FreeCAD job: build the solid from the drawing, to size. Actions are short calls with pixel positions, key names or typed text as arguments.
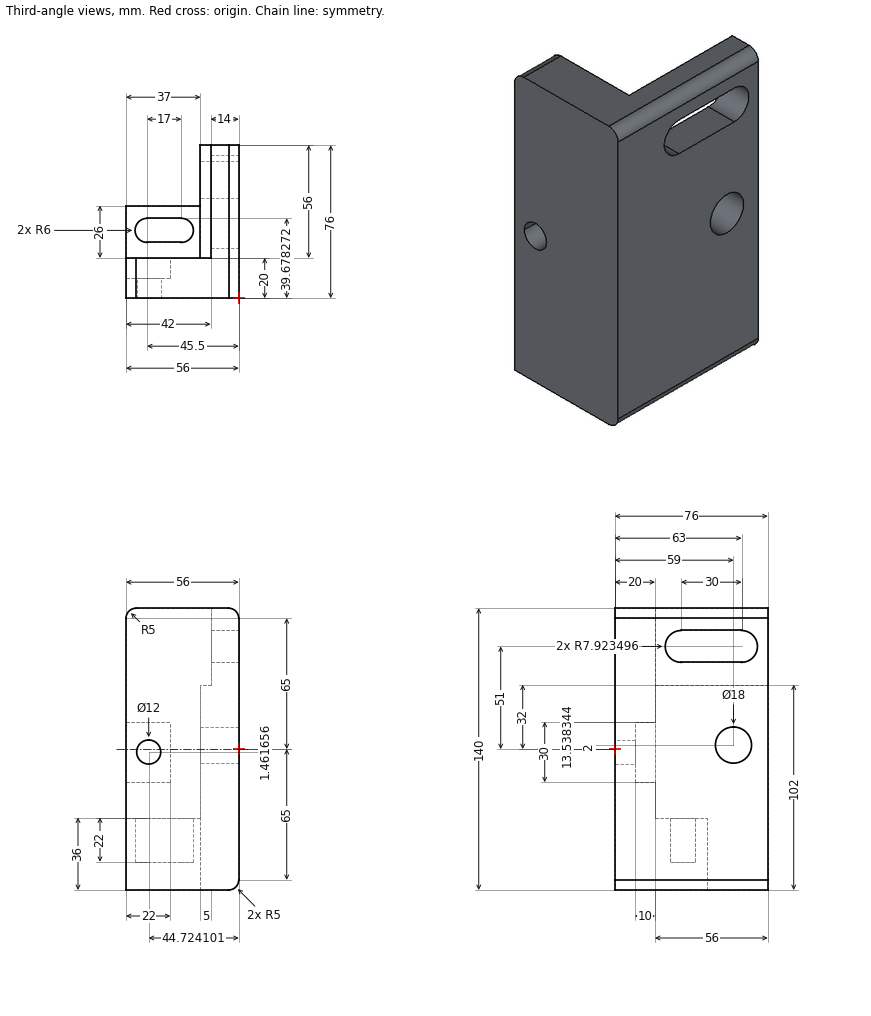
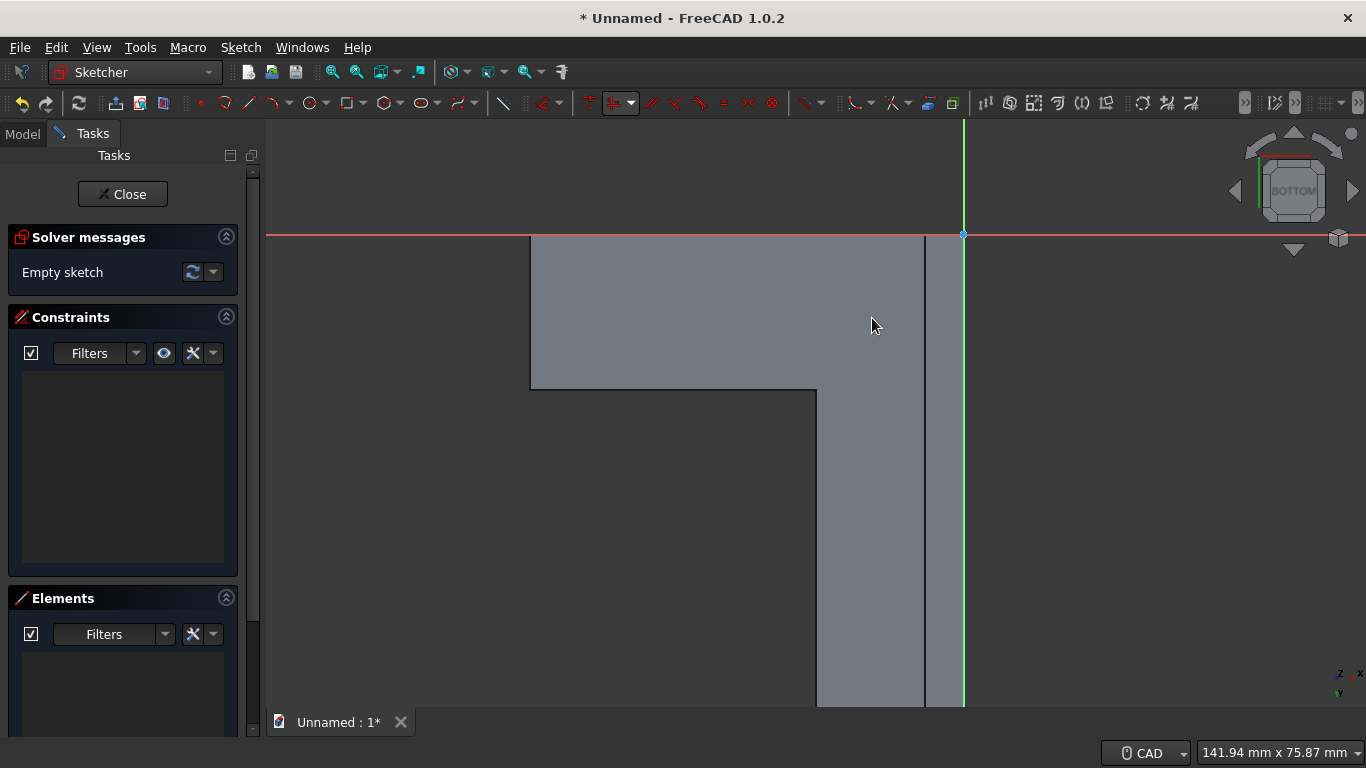
key(g)
key(r)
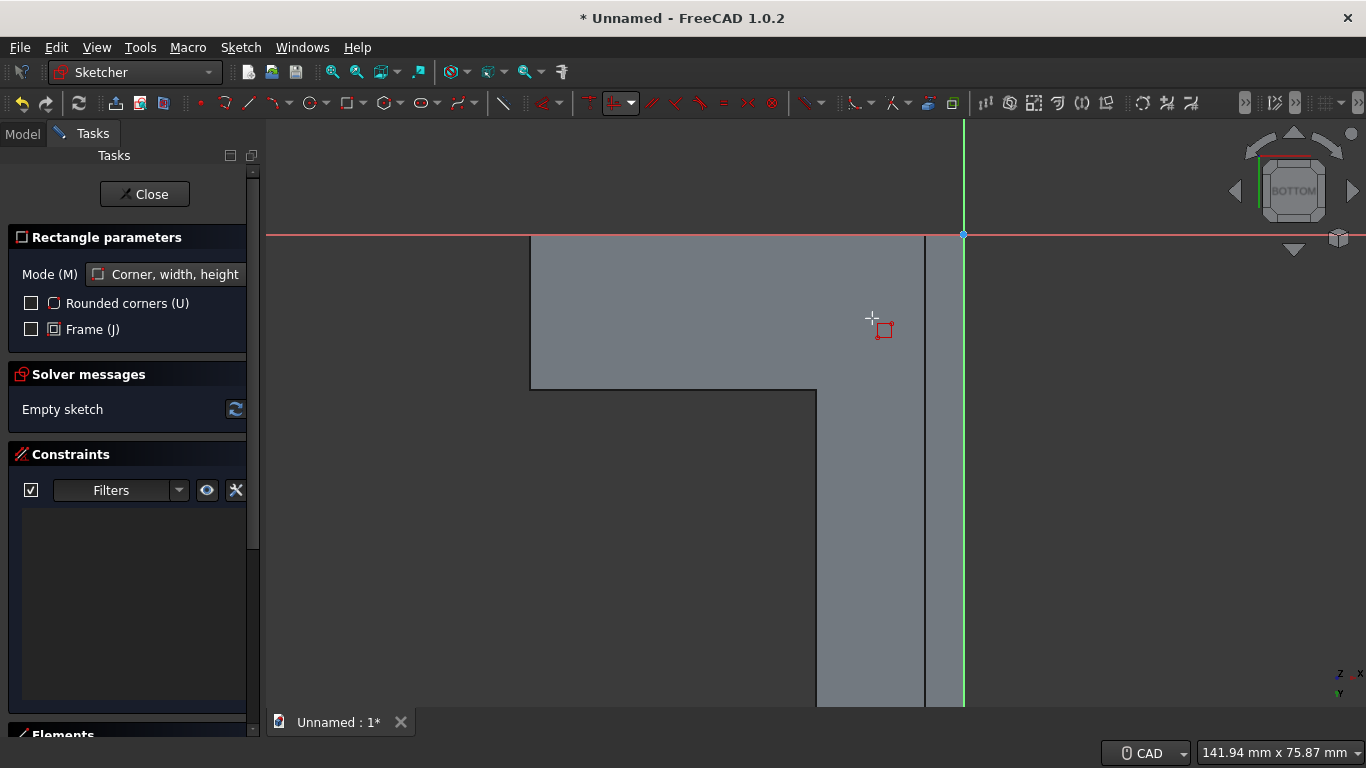
click(530, 390)
click(816, 591)
key(Escape)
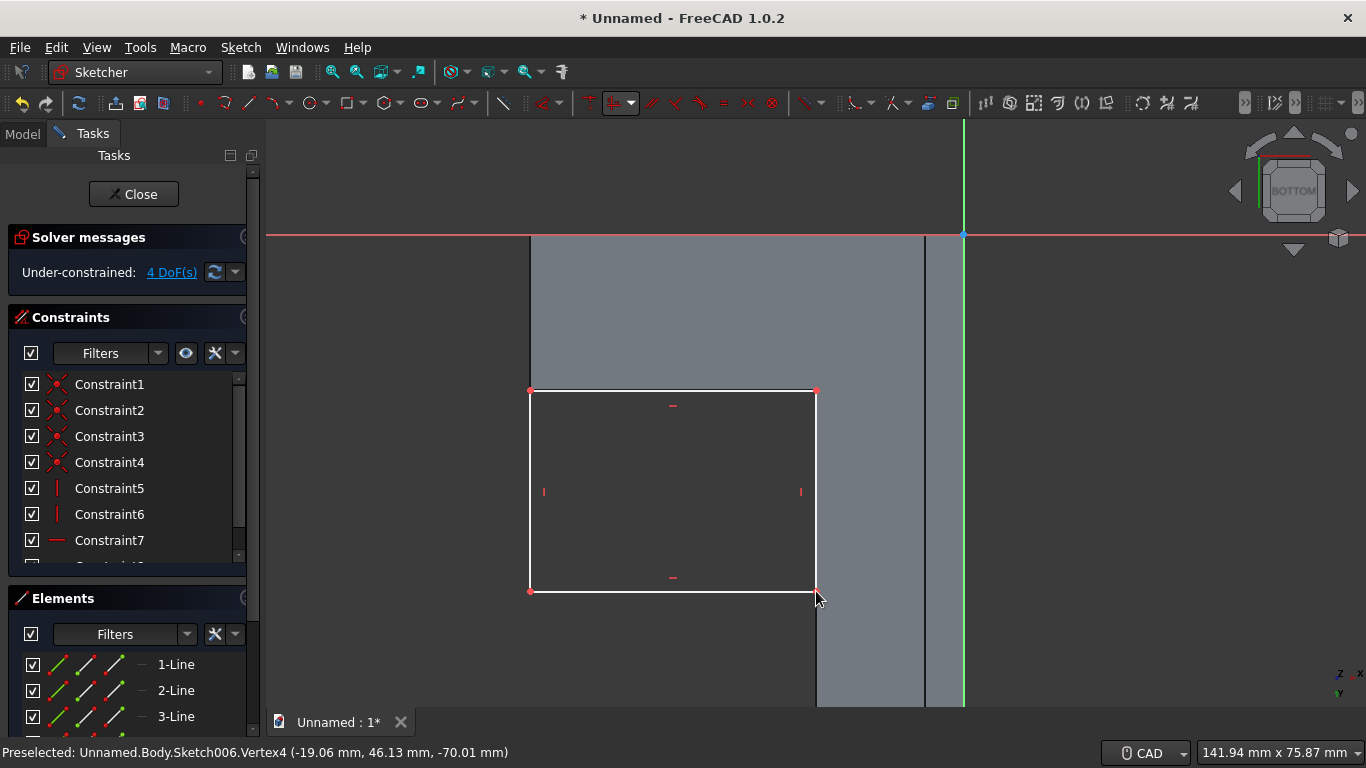
key(d)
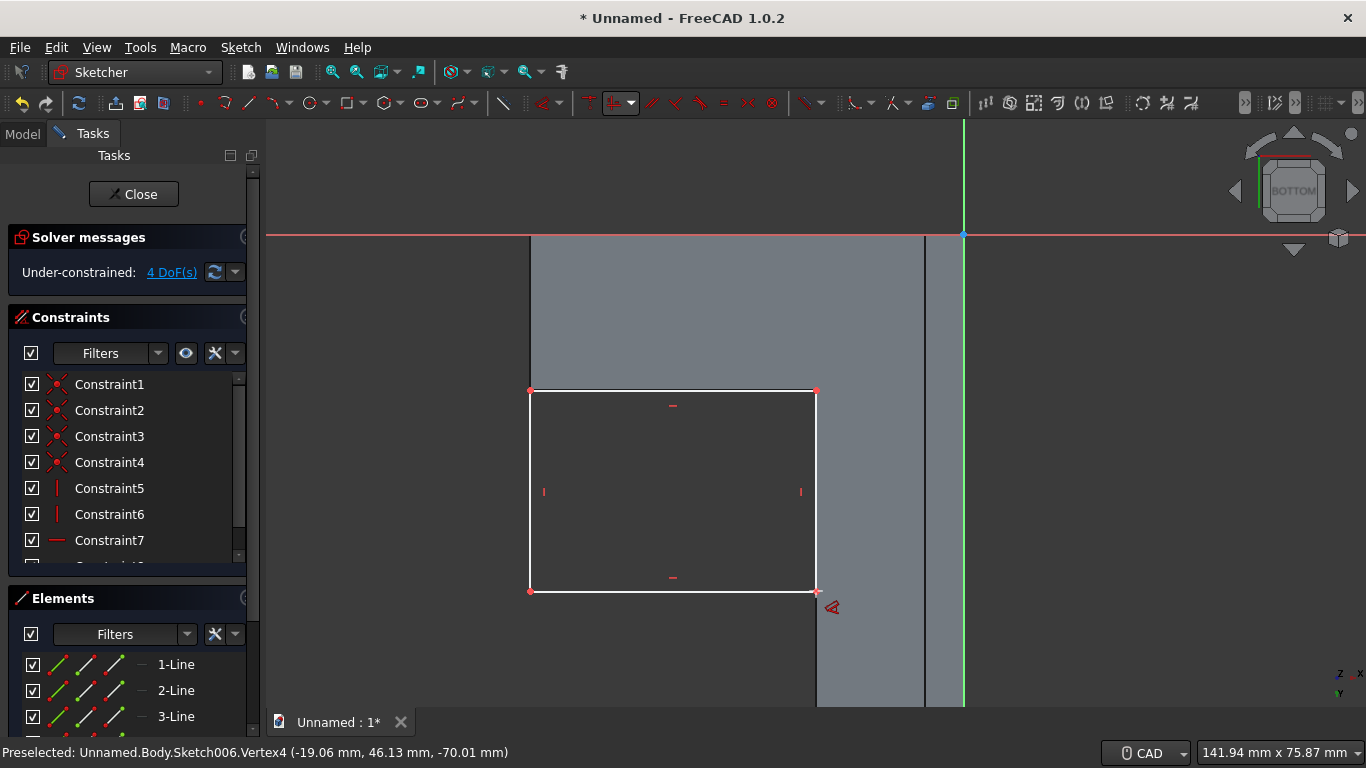
click(530, 451)
click(496, 491)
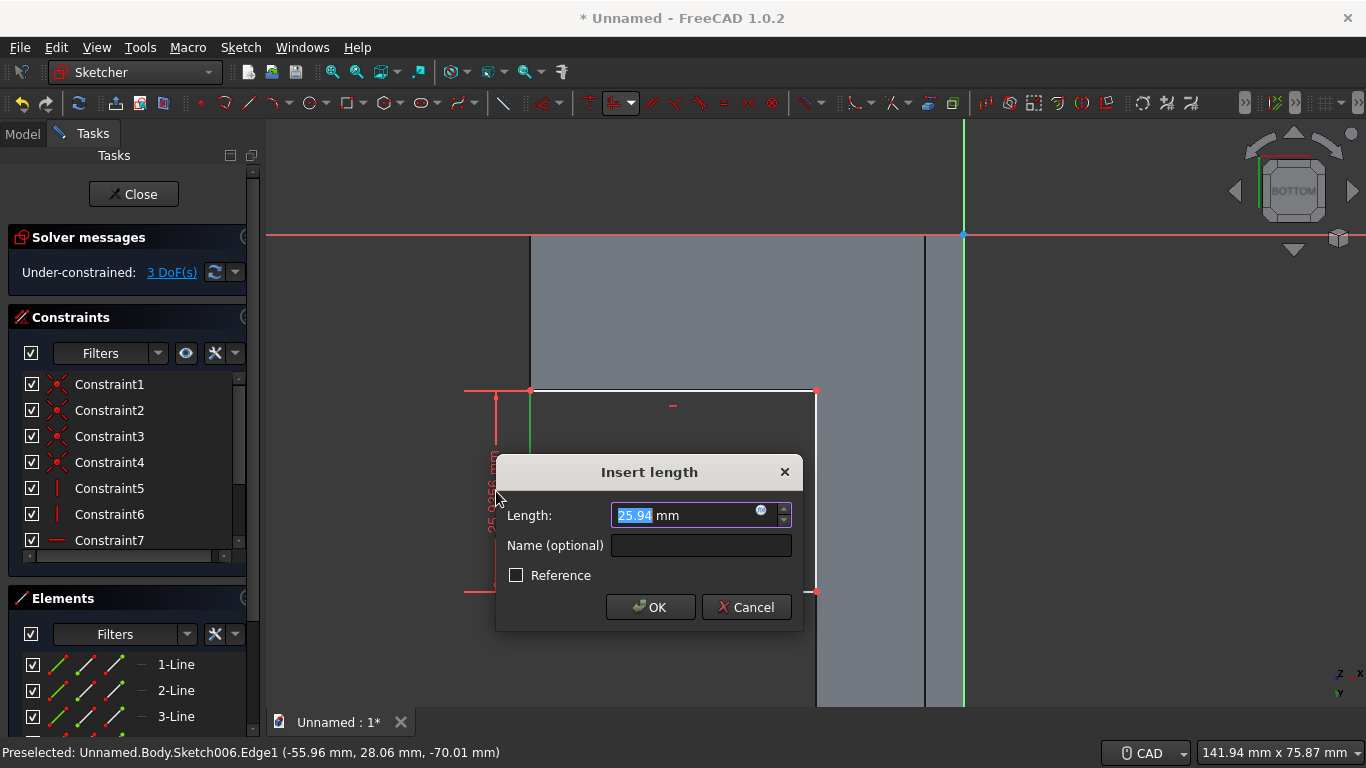
text(26)
key(Return)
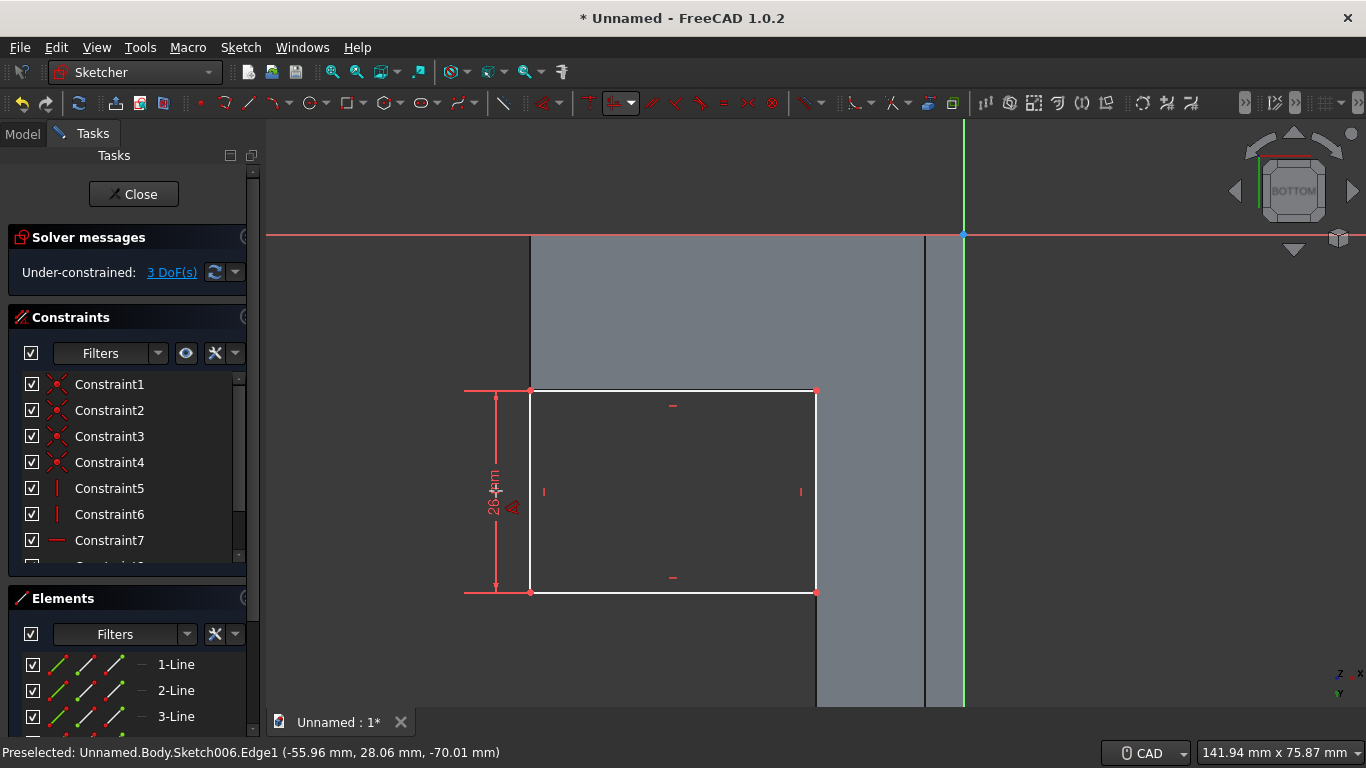
click(616, 592)
click(673, 626)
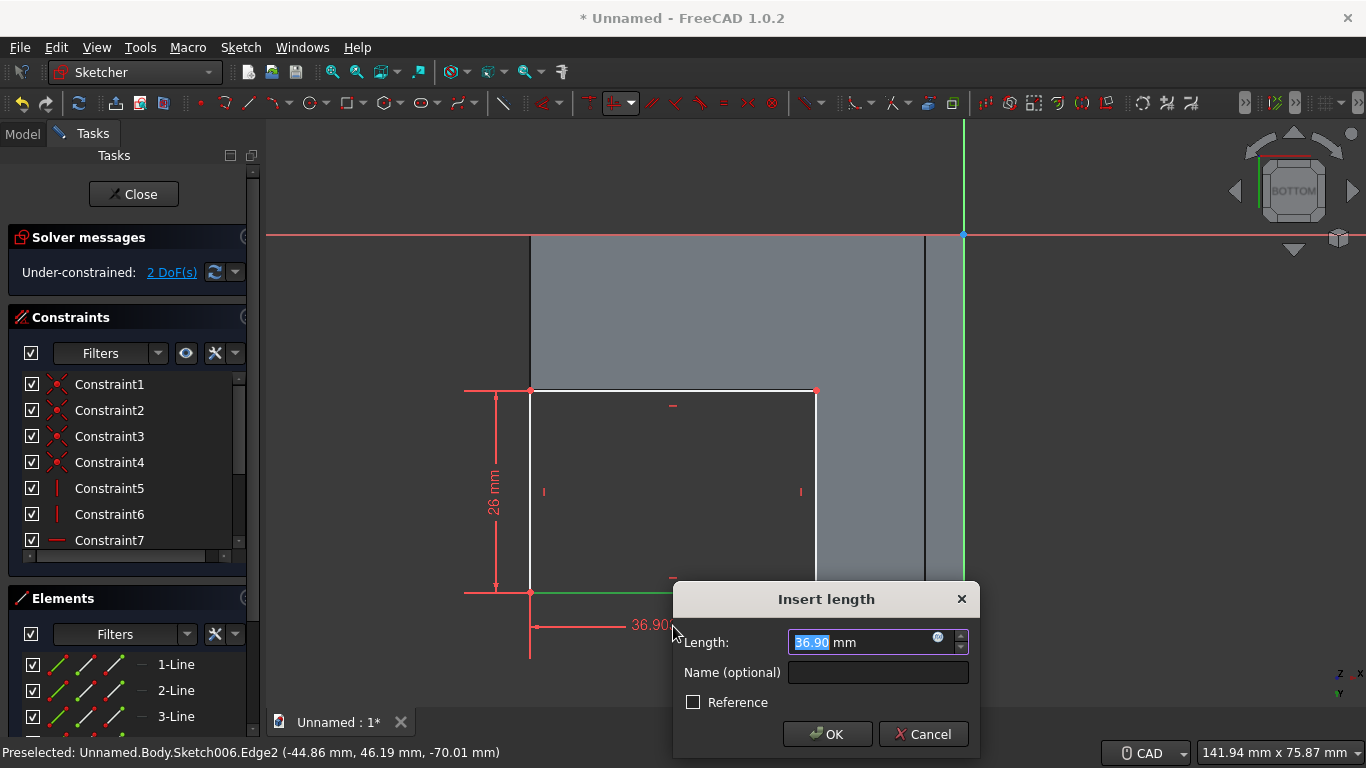
text(37)
key(Return)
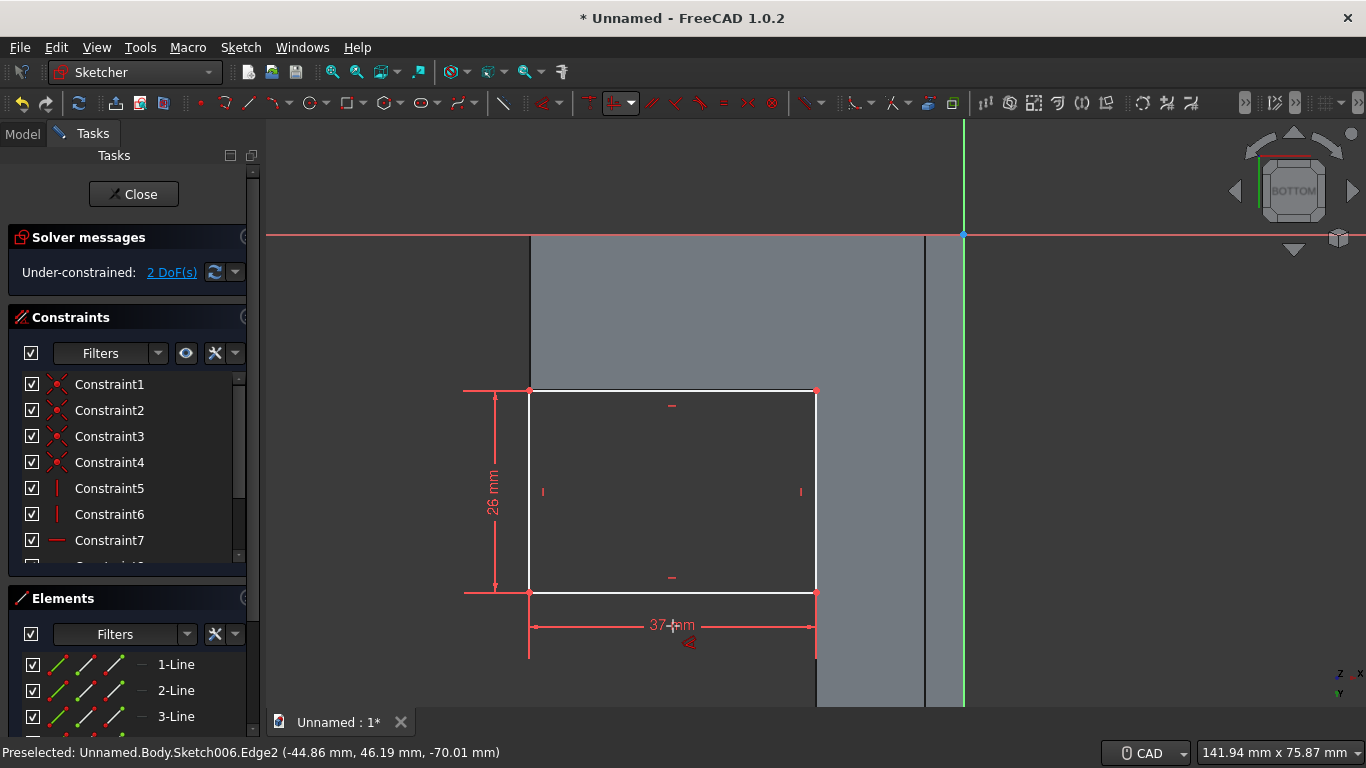
click(529, 391)
click(746, 201)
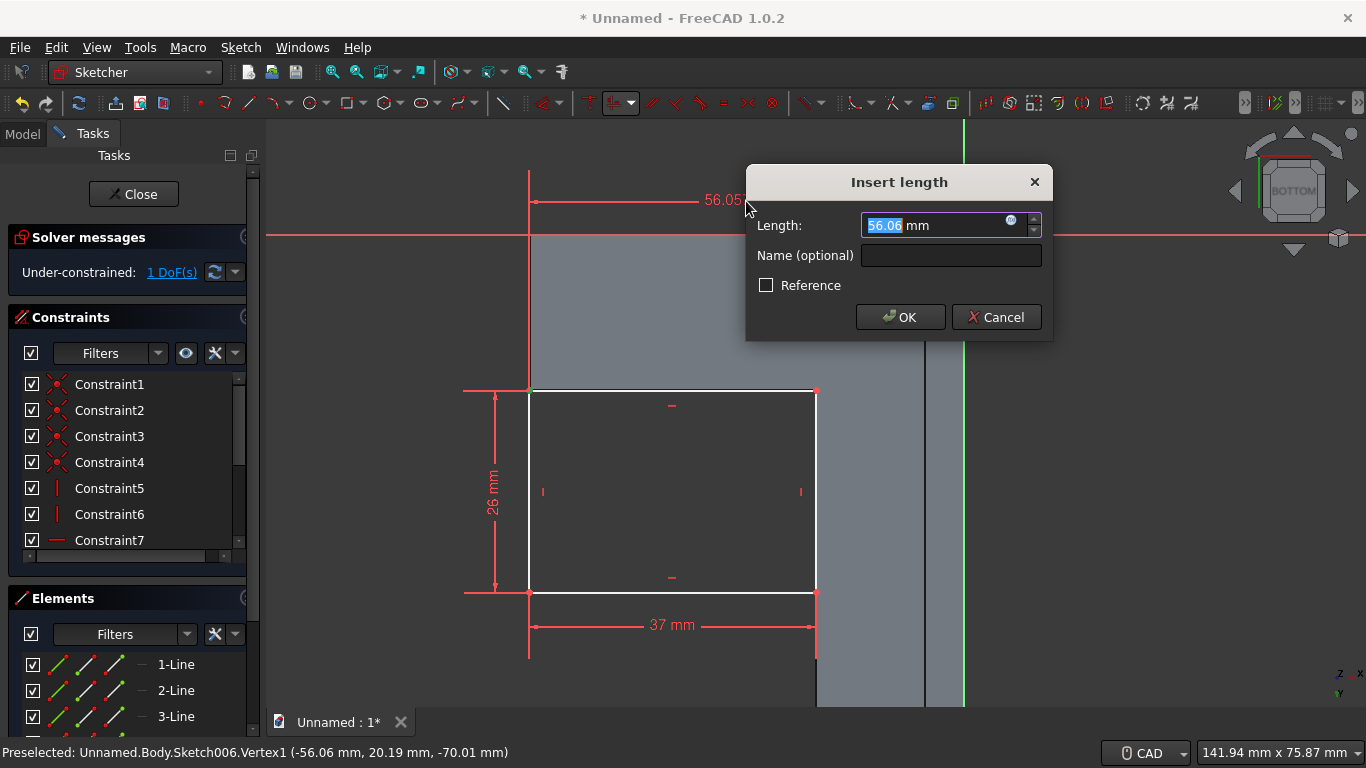
text(56)
key(Return)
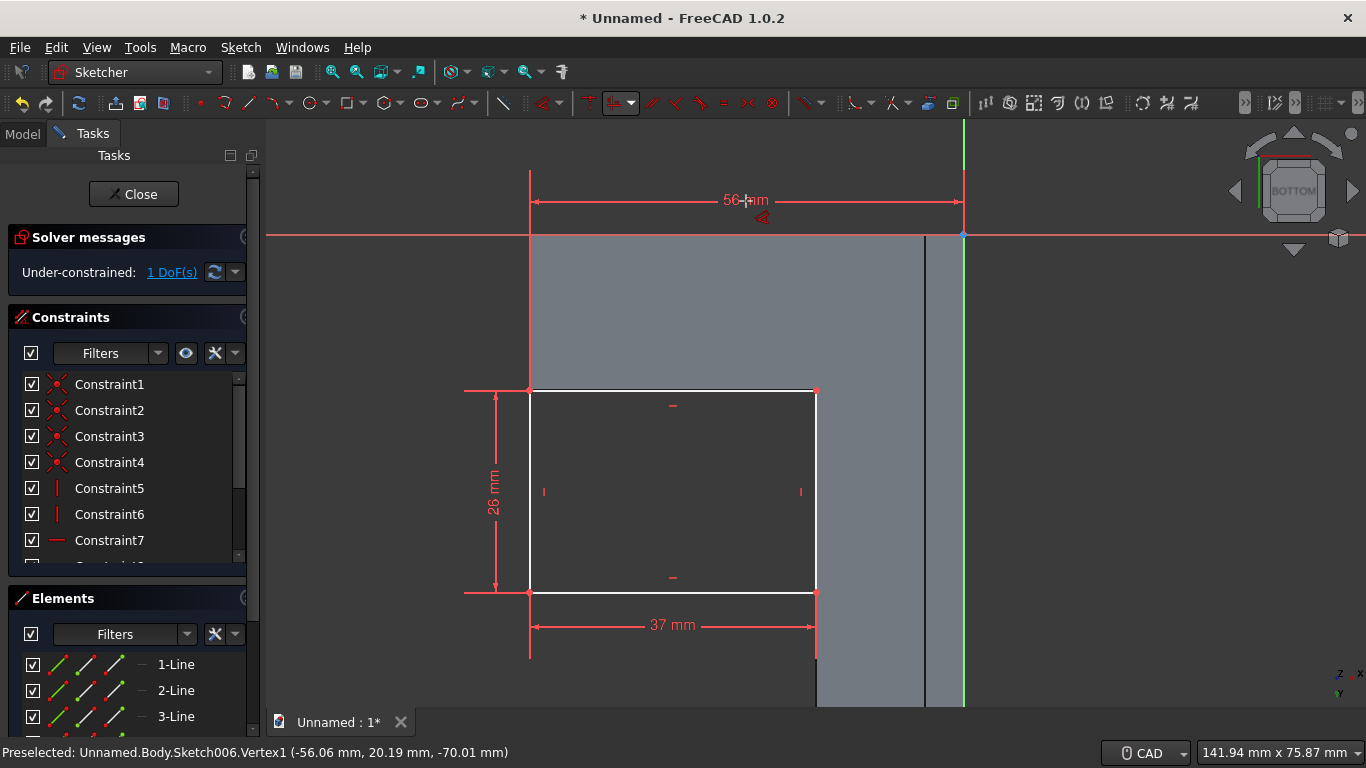
click(530, 391)
click(998, 313)